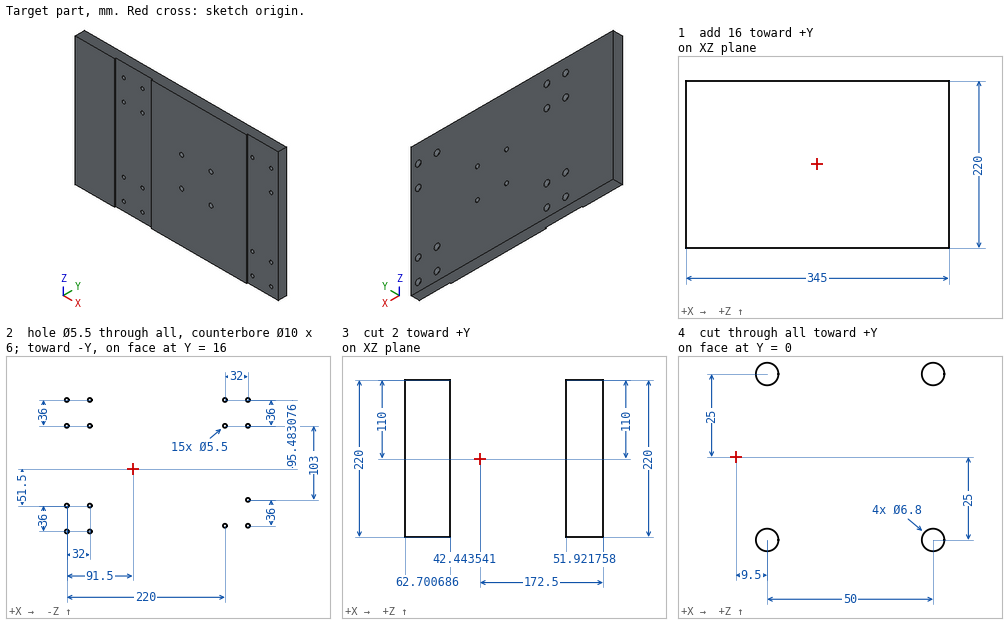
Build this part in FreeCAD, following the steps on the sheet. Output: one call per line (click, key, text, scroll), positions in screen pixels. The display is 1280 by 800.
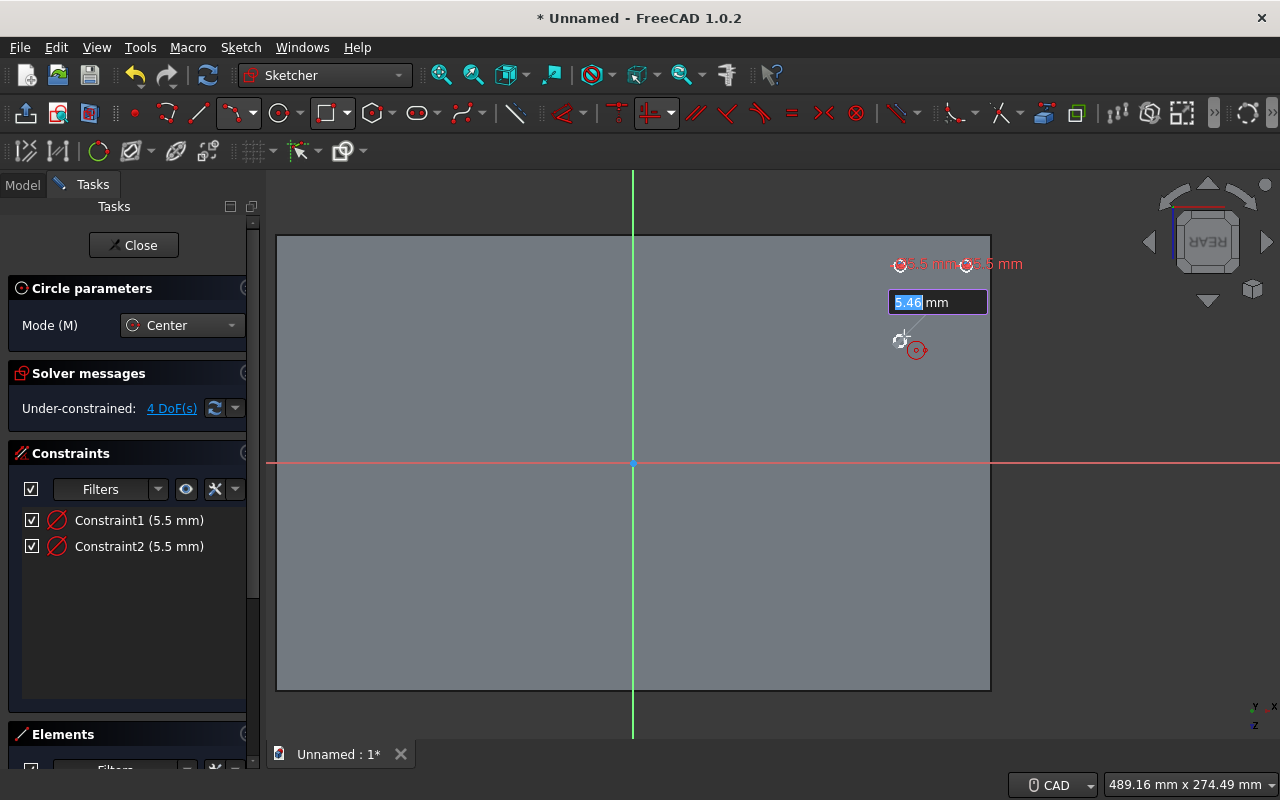
text(5.5)
key(Return)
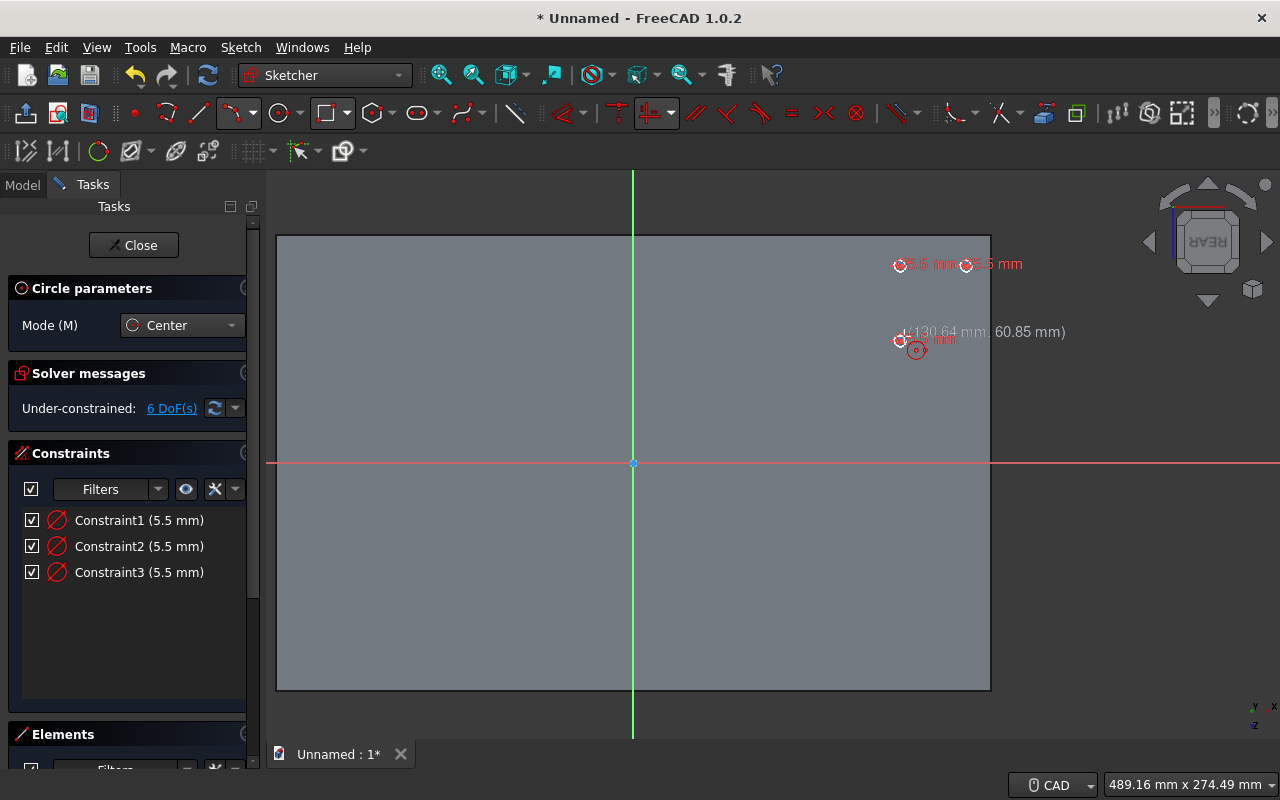
scroll(966, 340, up, 7)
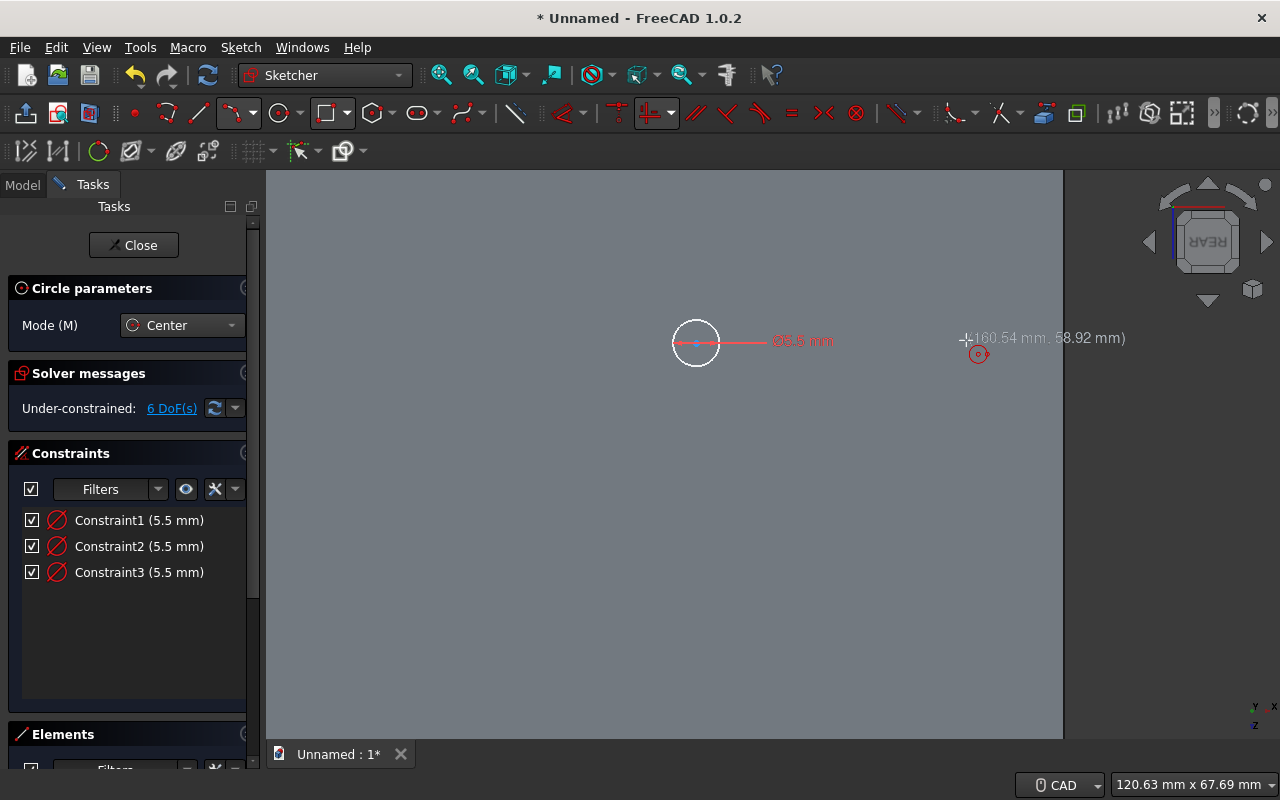
scroll(966, 340, down, 7)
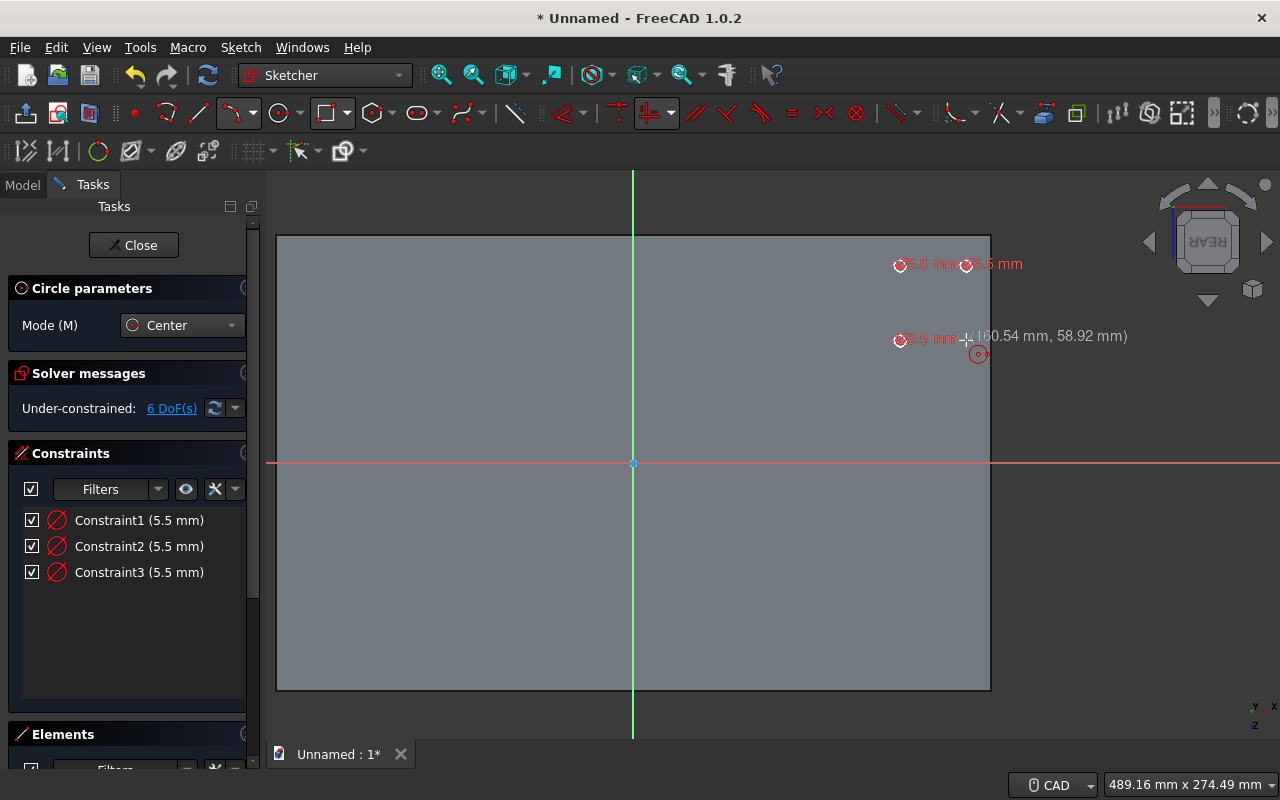
click(966, 340)
move(970, 336)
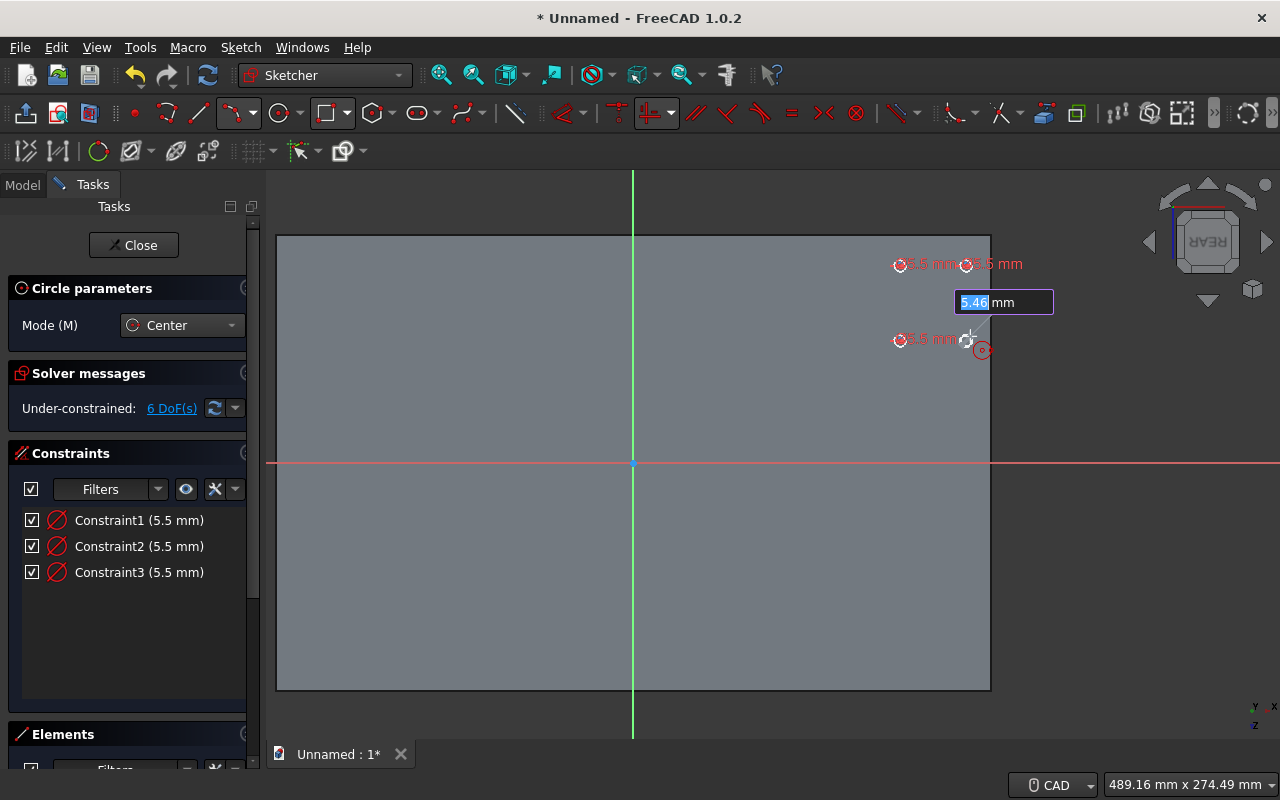
text(5.5)
key(Return)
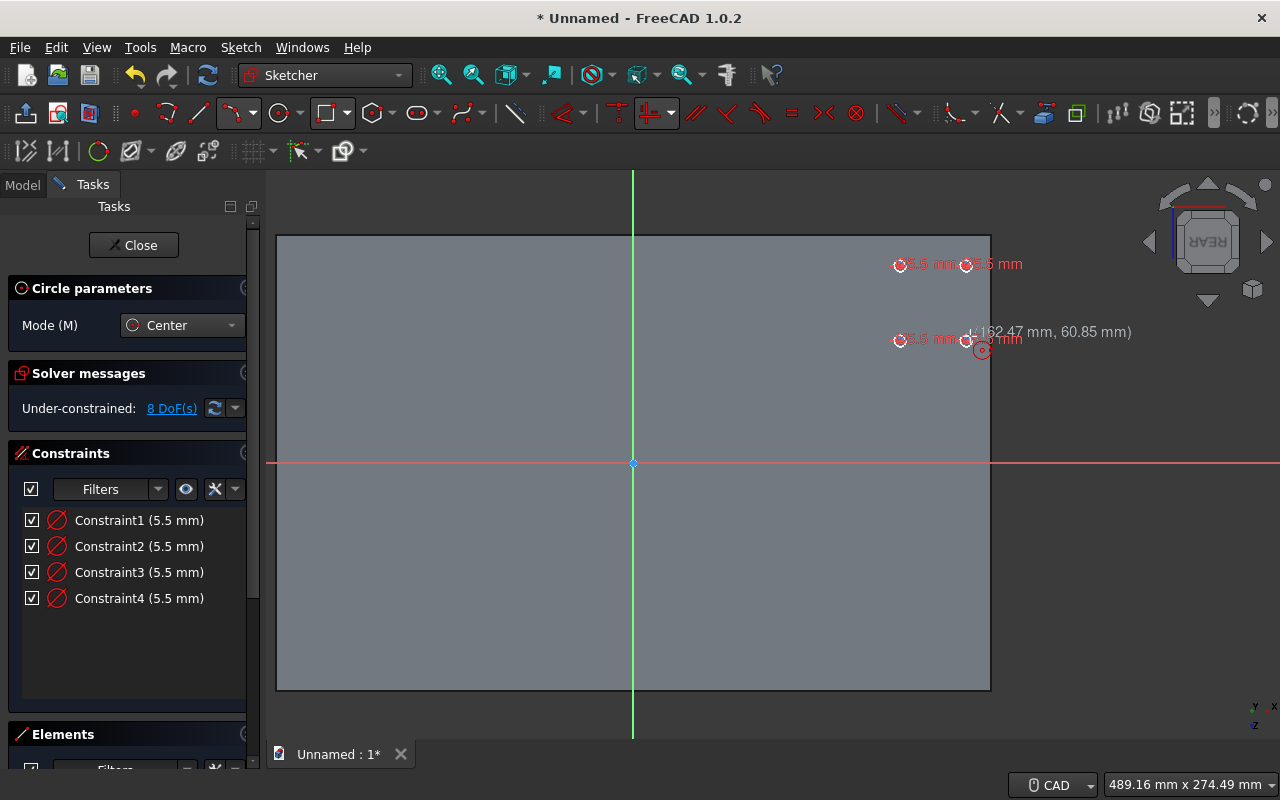
scroll(966, 553, up, 7)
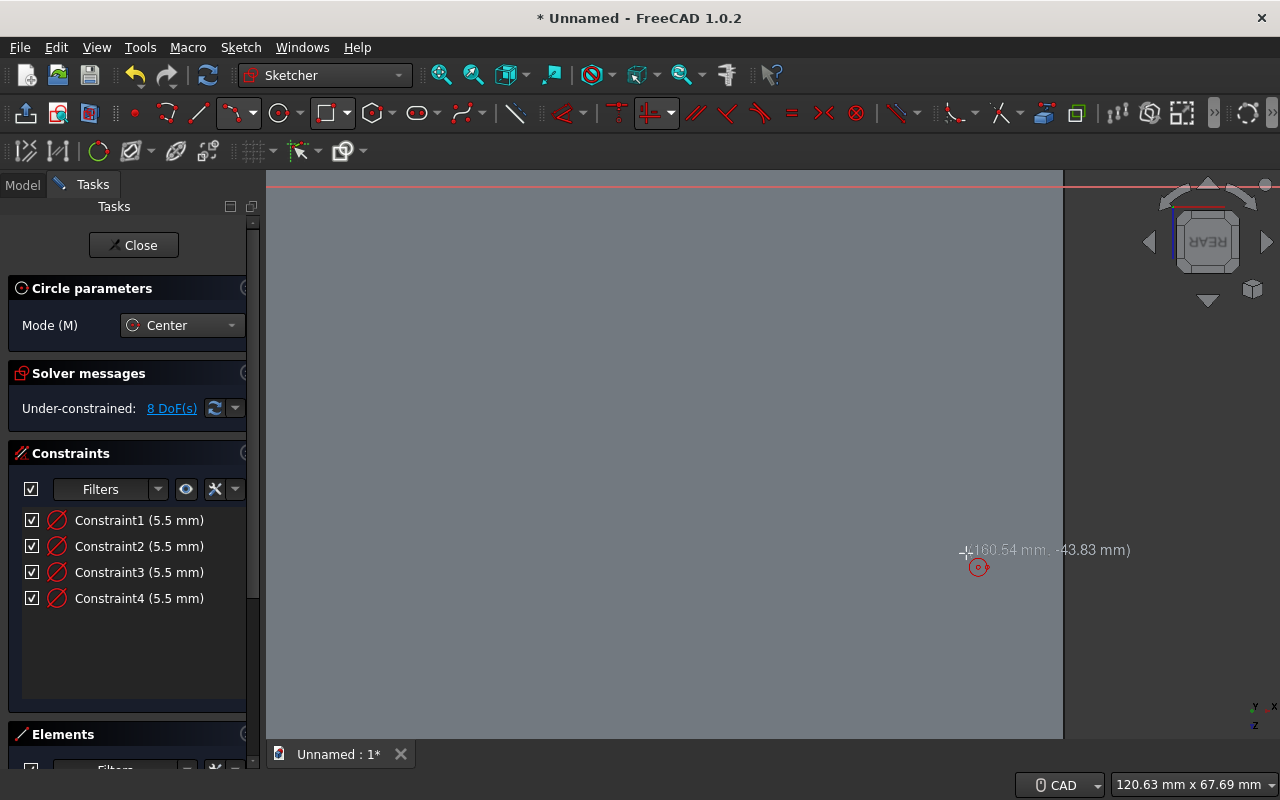
scroll(966, 553, down, 7)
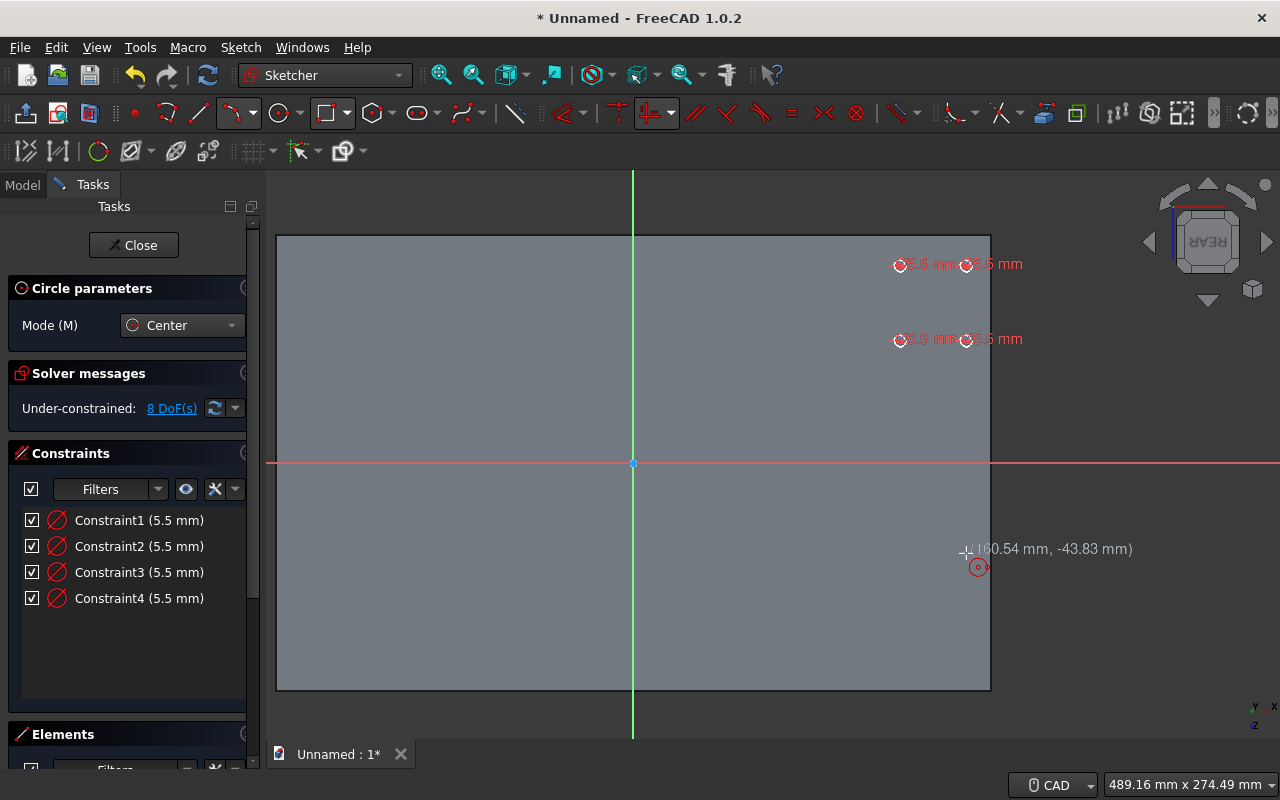
click(966, 553)
move(970, 549)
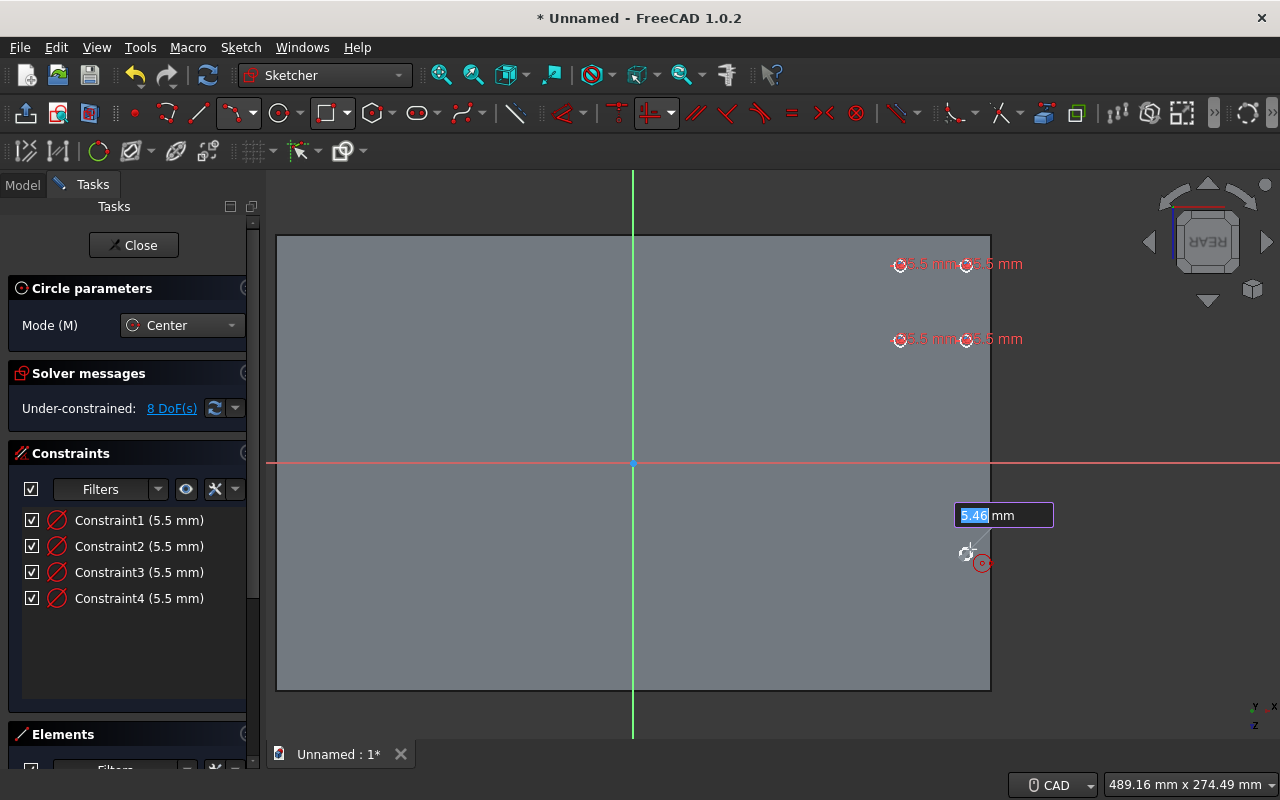
text(5.5)
key(Return)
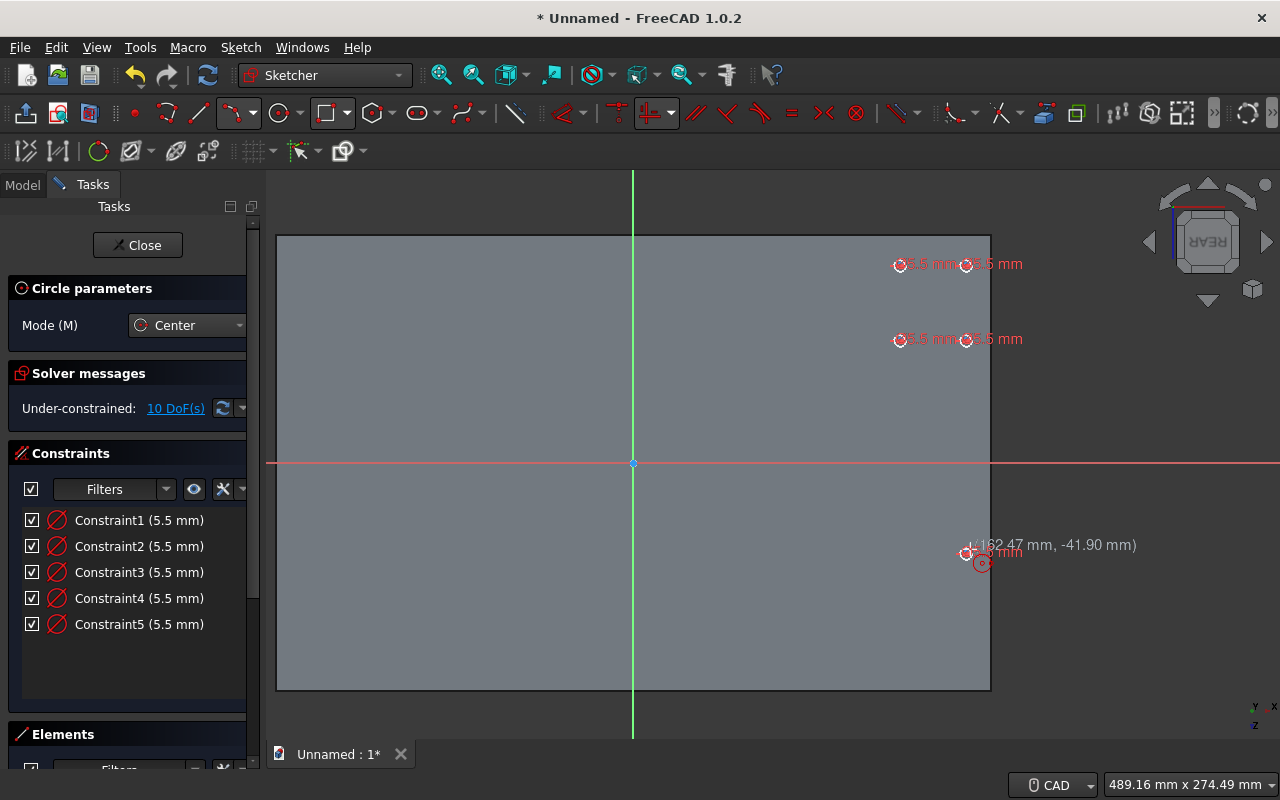
scroll(966, 628, up, 7)